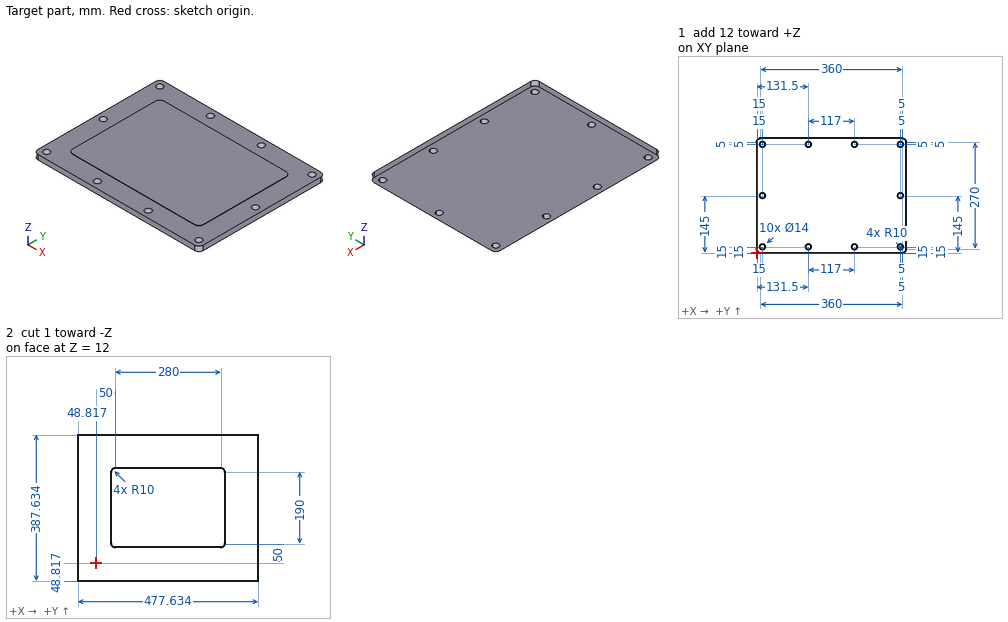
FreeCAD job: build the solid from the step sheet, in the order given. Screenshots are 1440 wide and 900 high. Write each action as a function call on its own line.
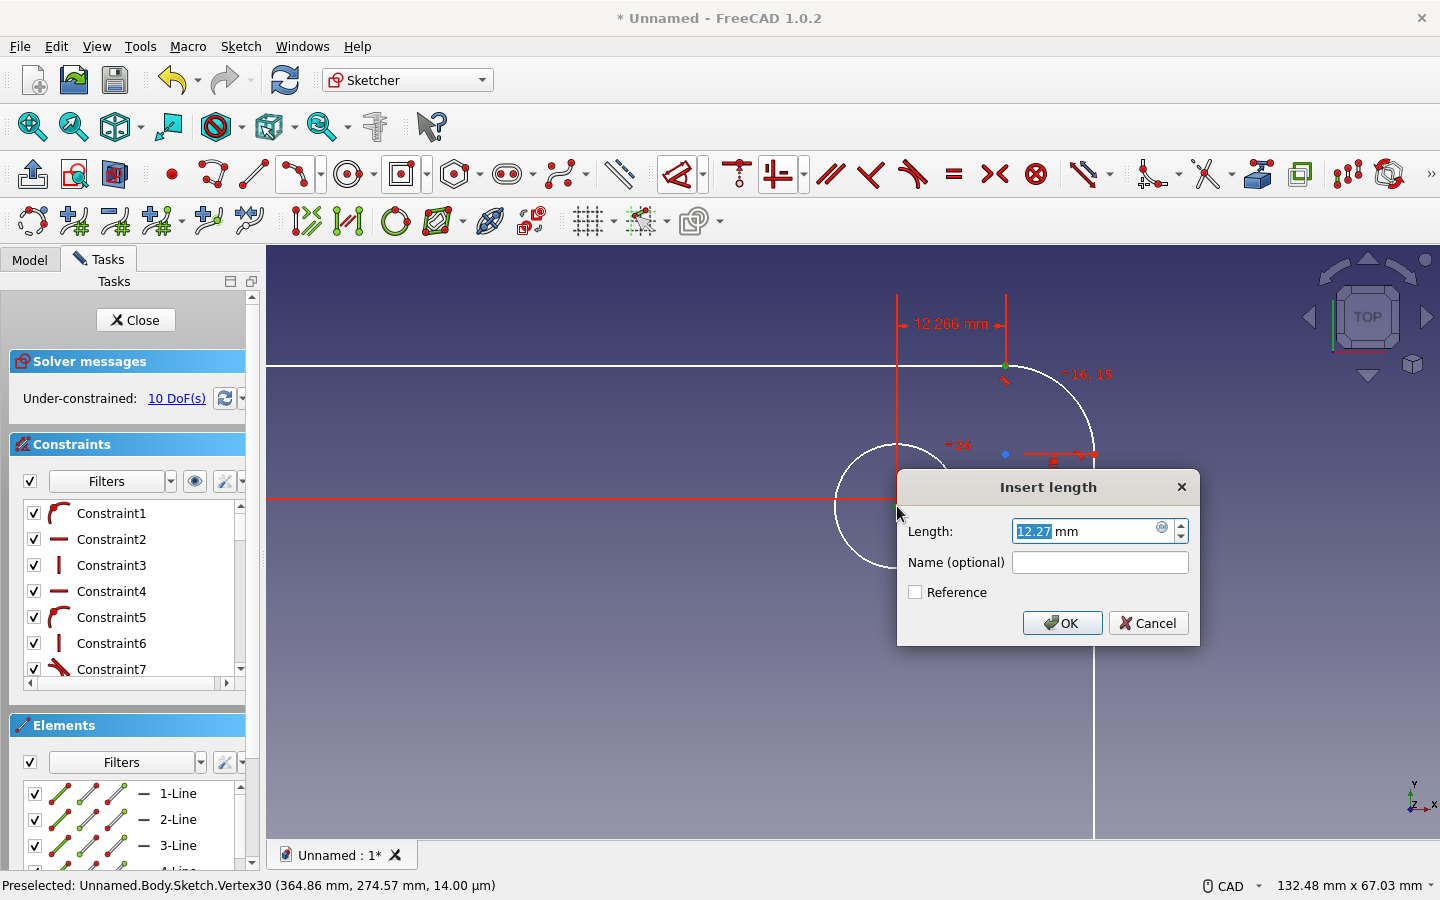
text(5)
key(Return)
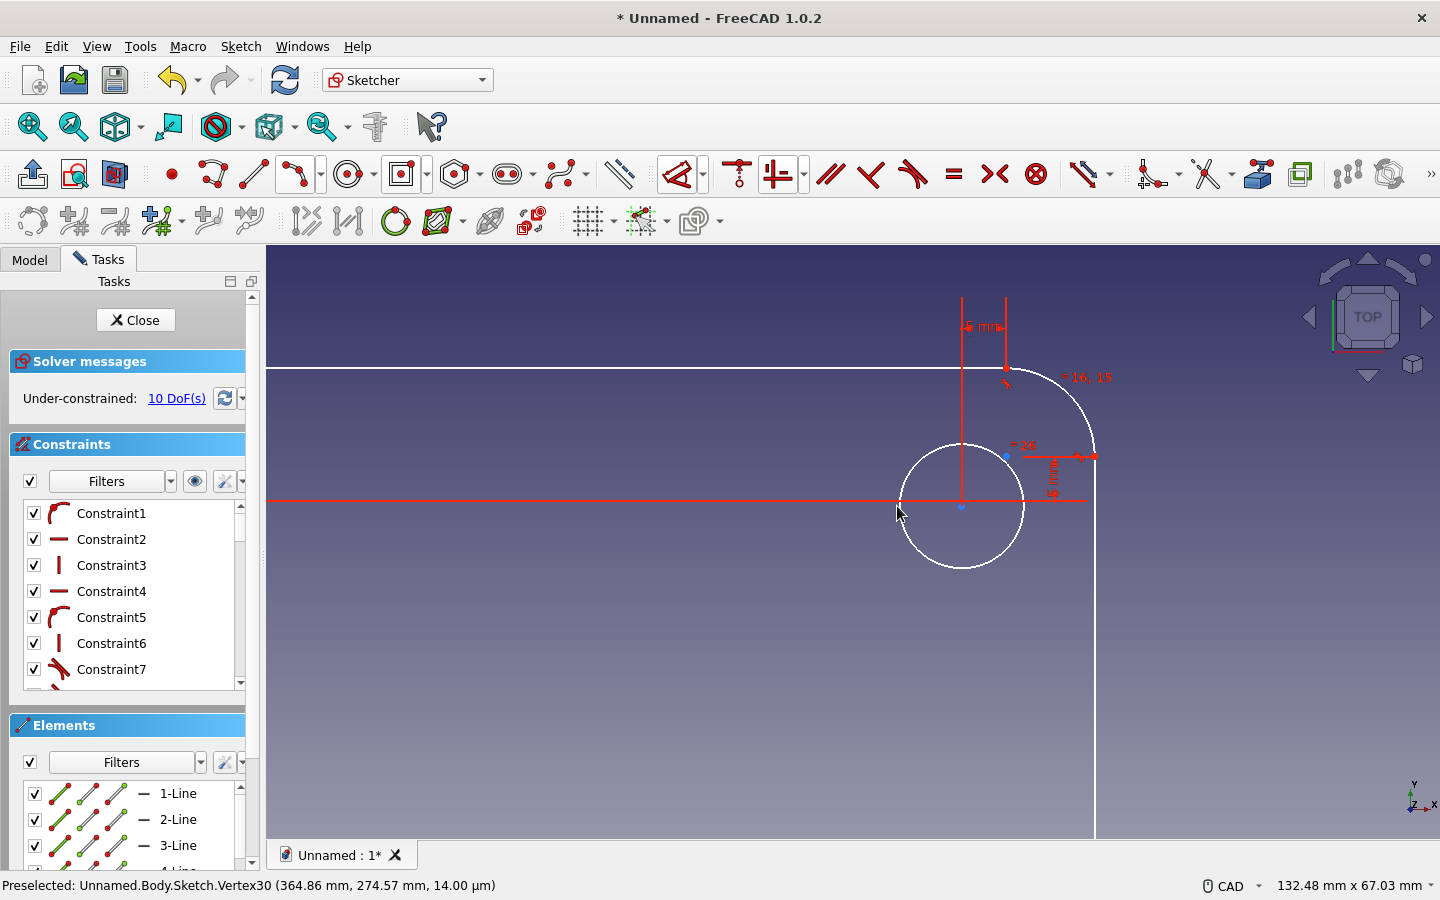
click(1095, 457)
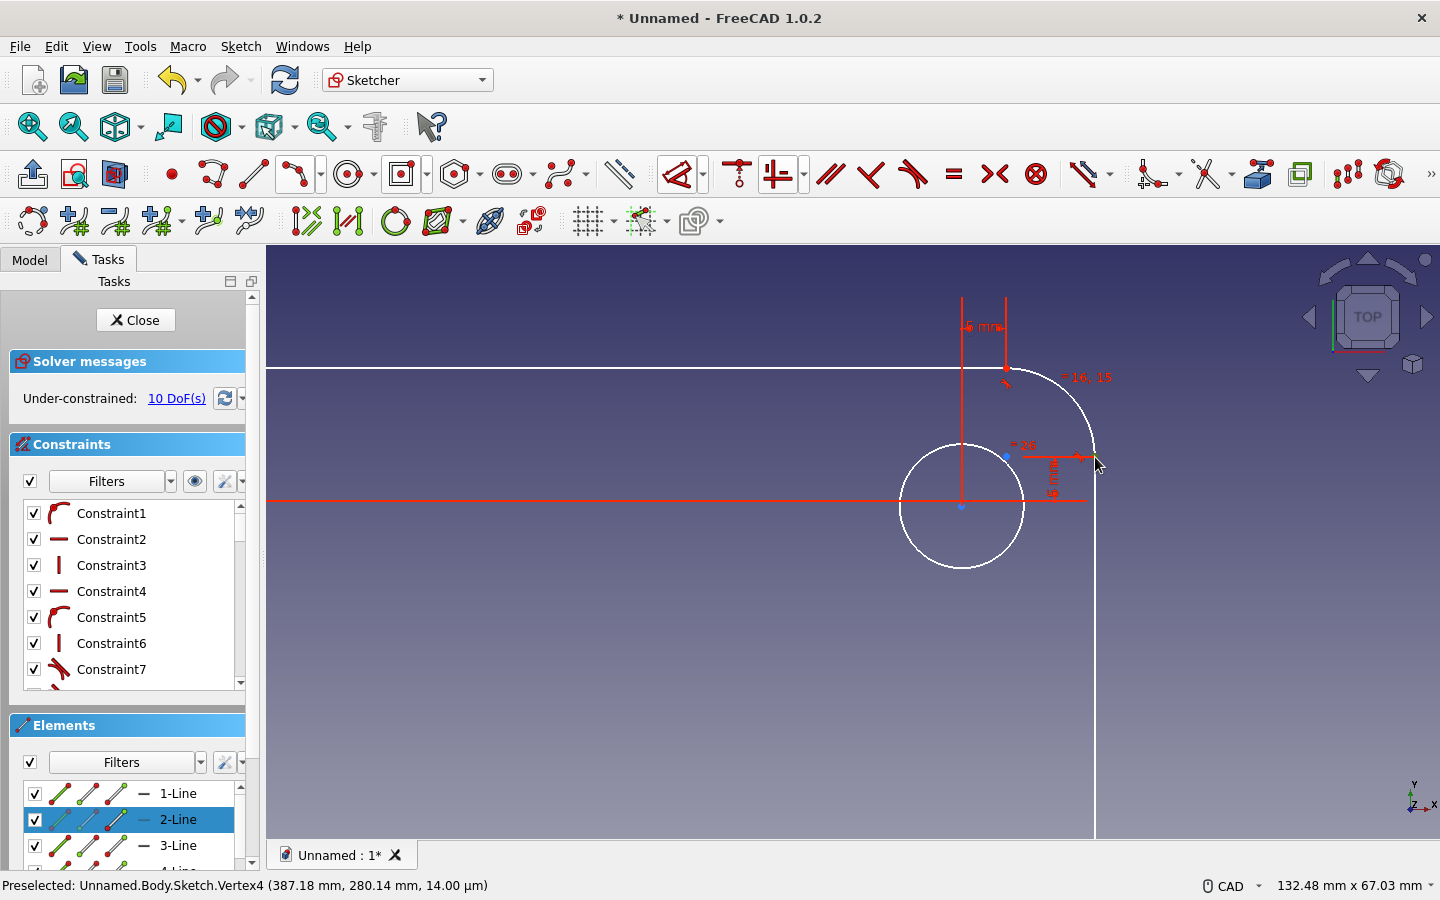
click(962, 506)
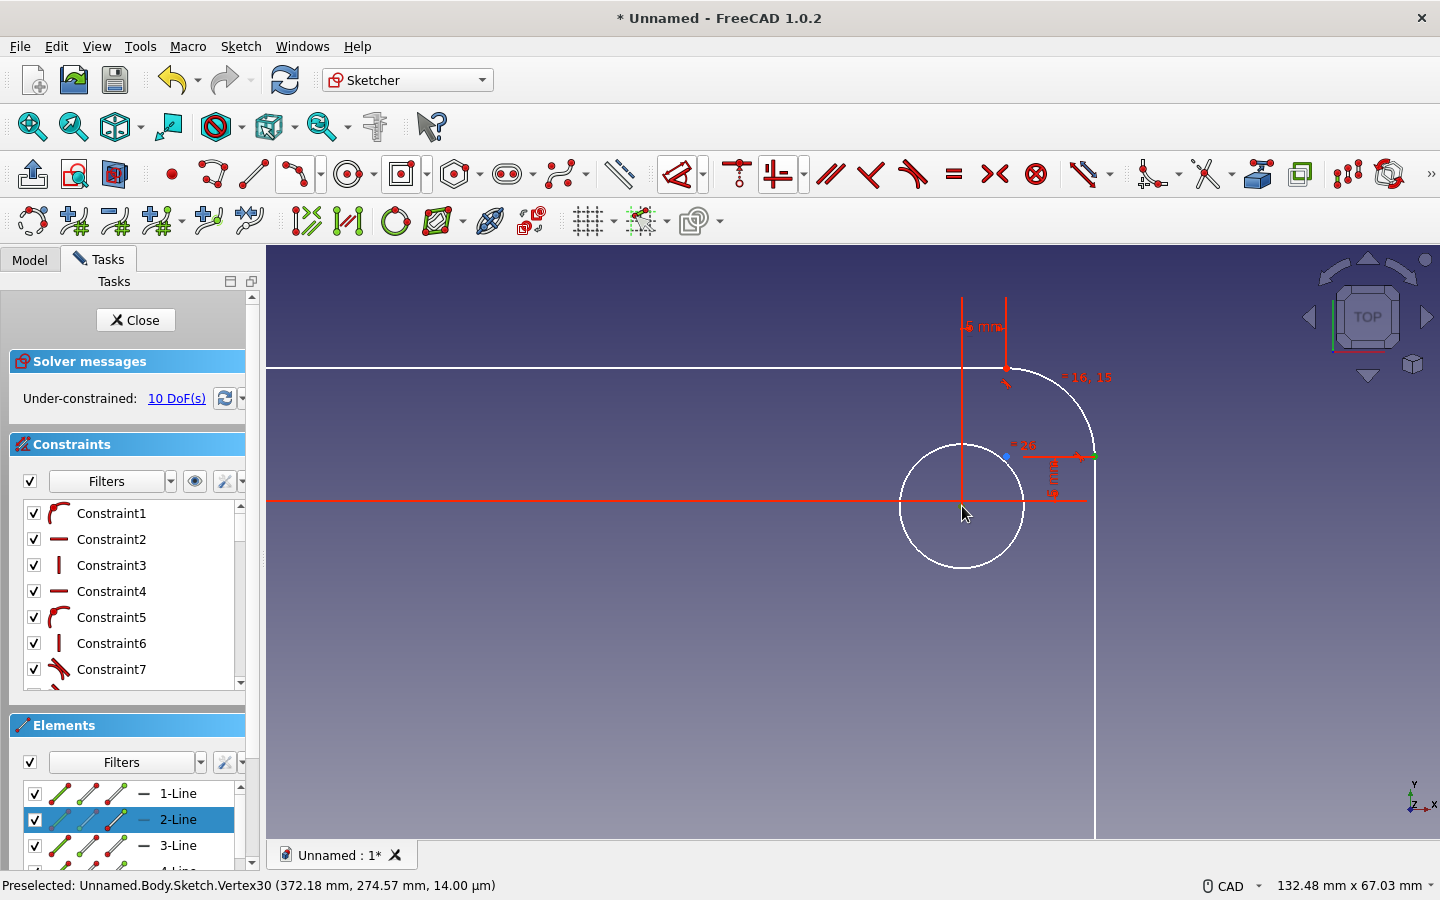
click(702, 174)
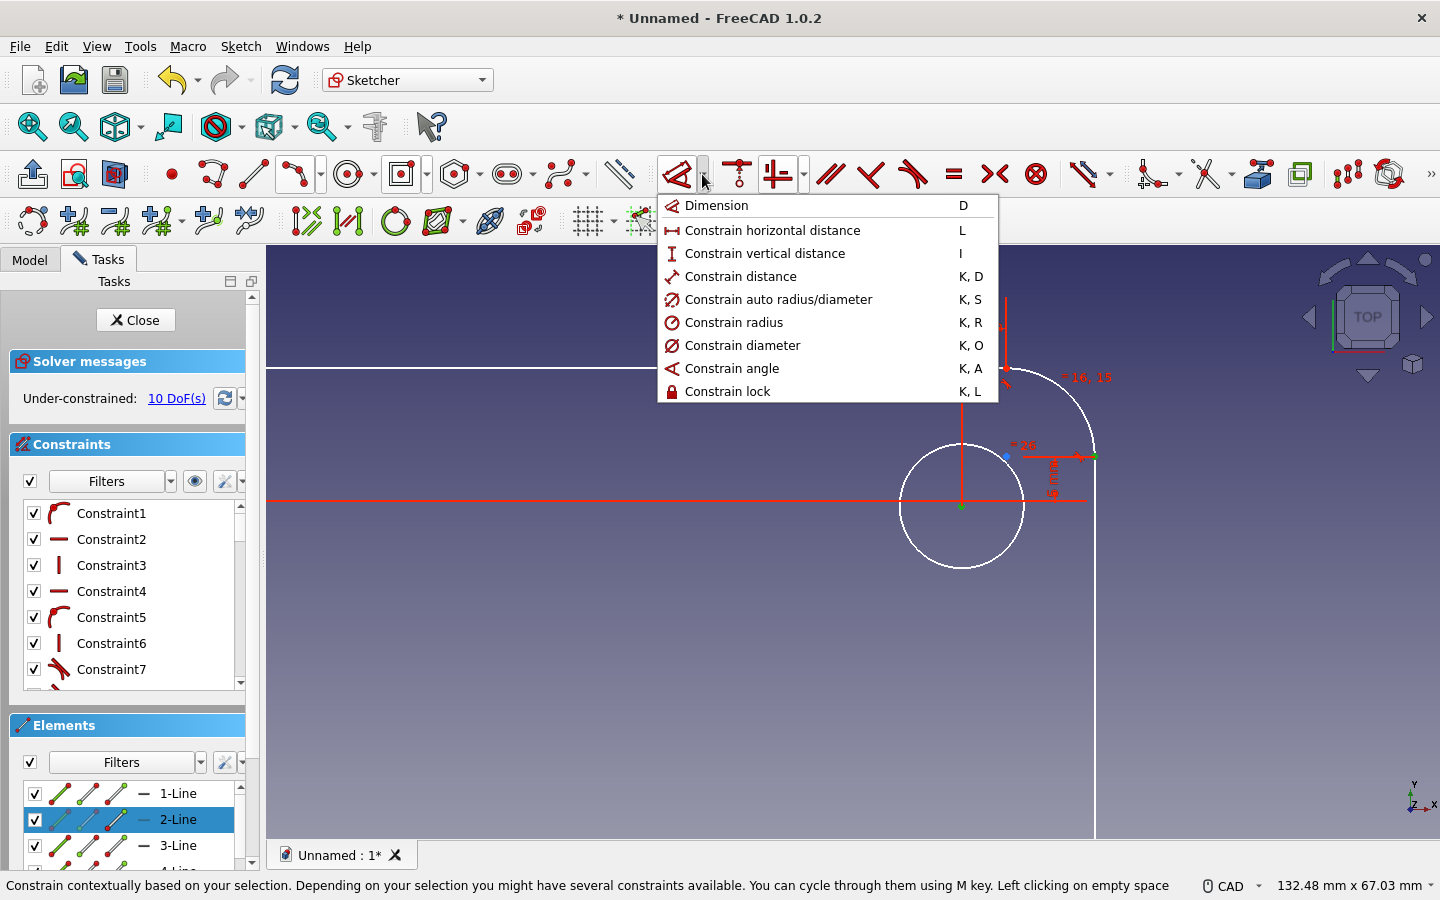
click(828, 254)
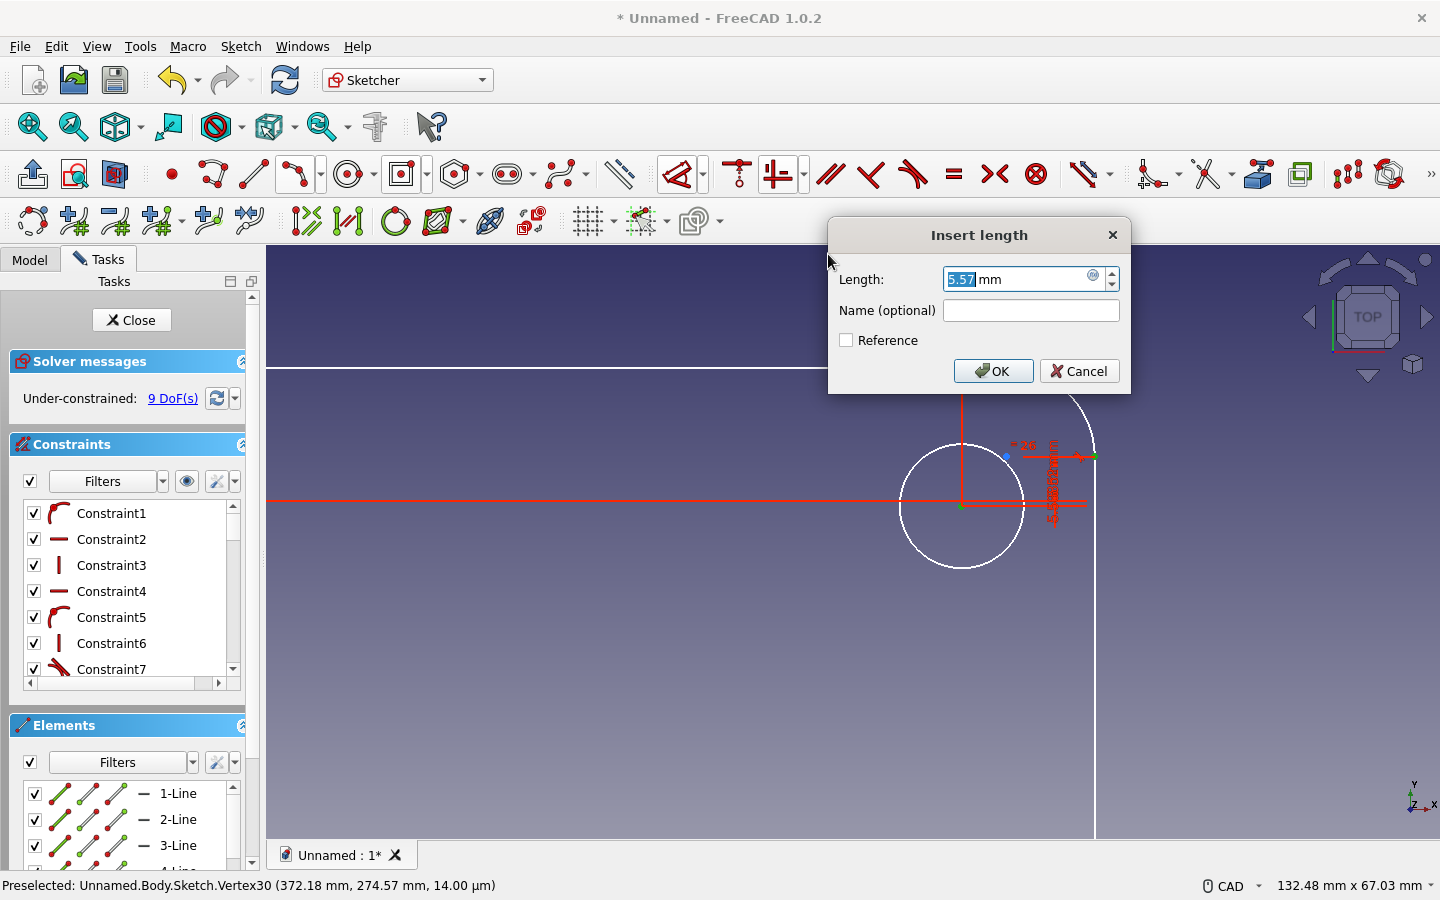
text(5)
key(Return)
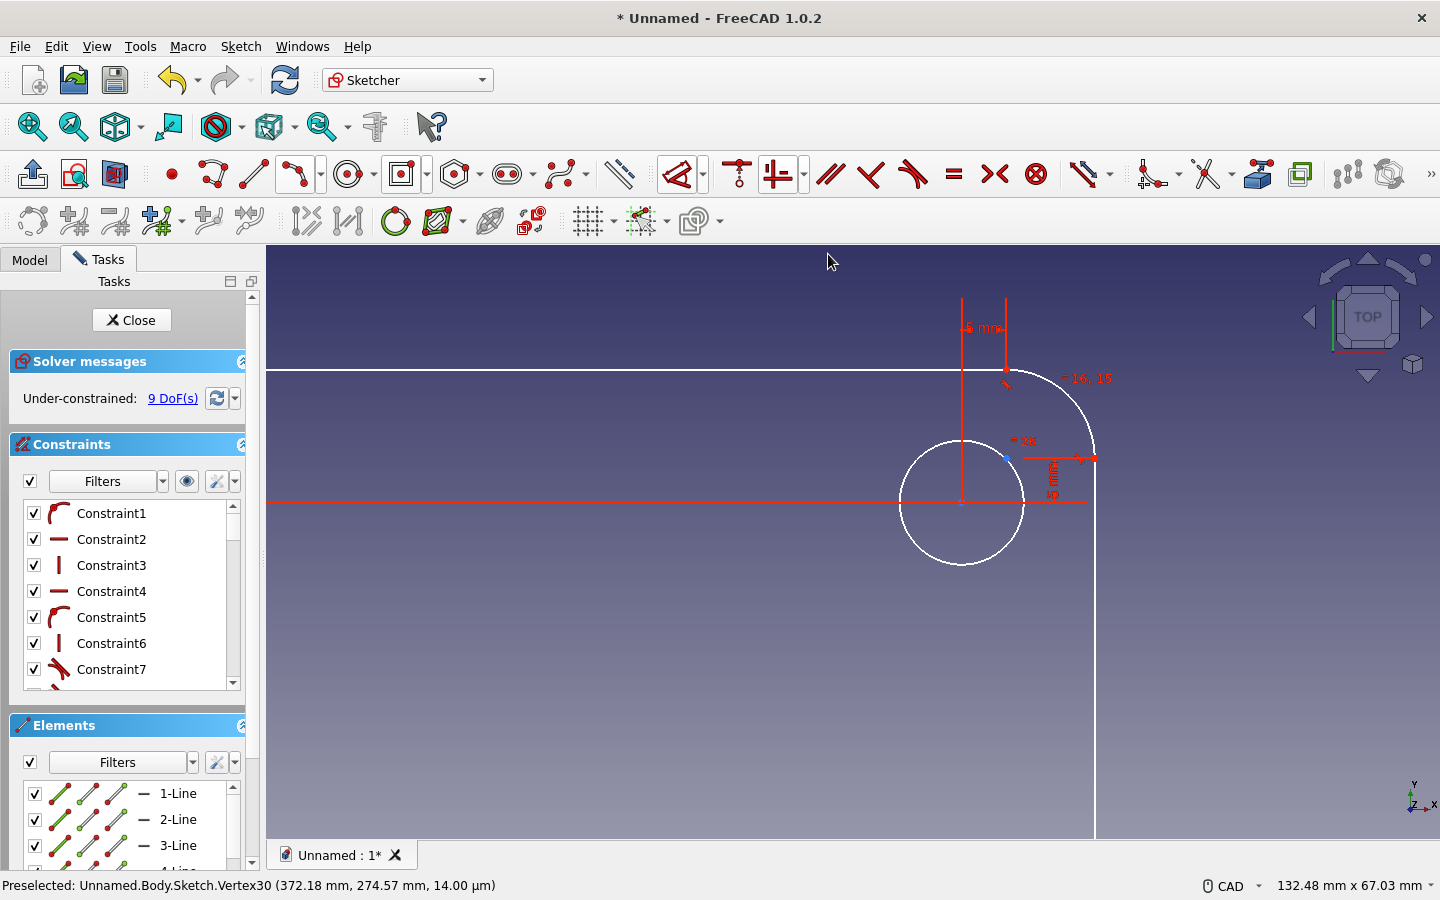
scroll(1009, 368, down, 10)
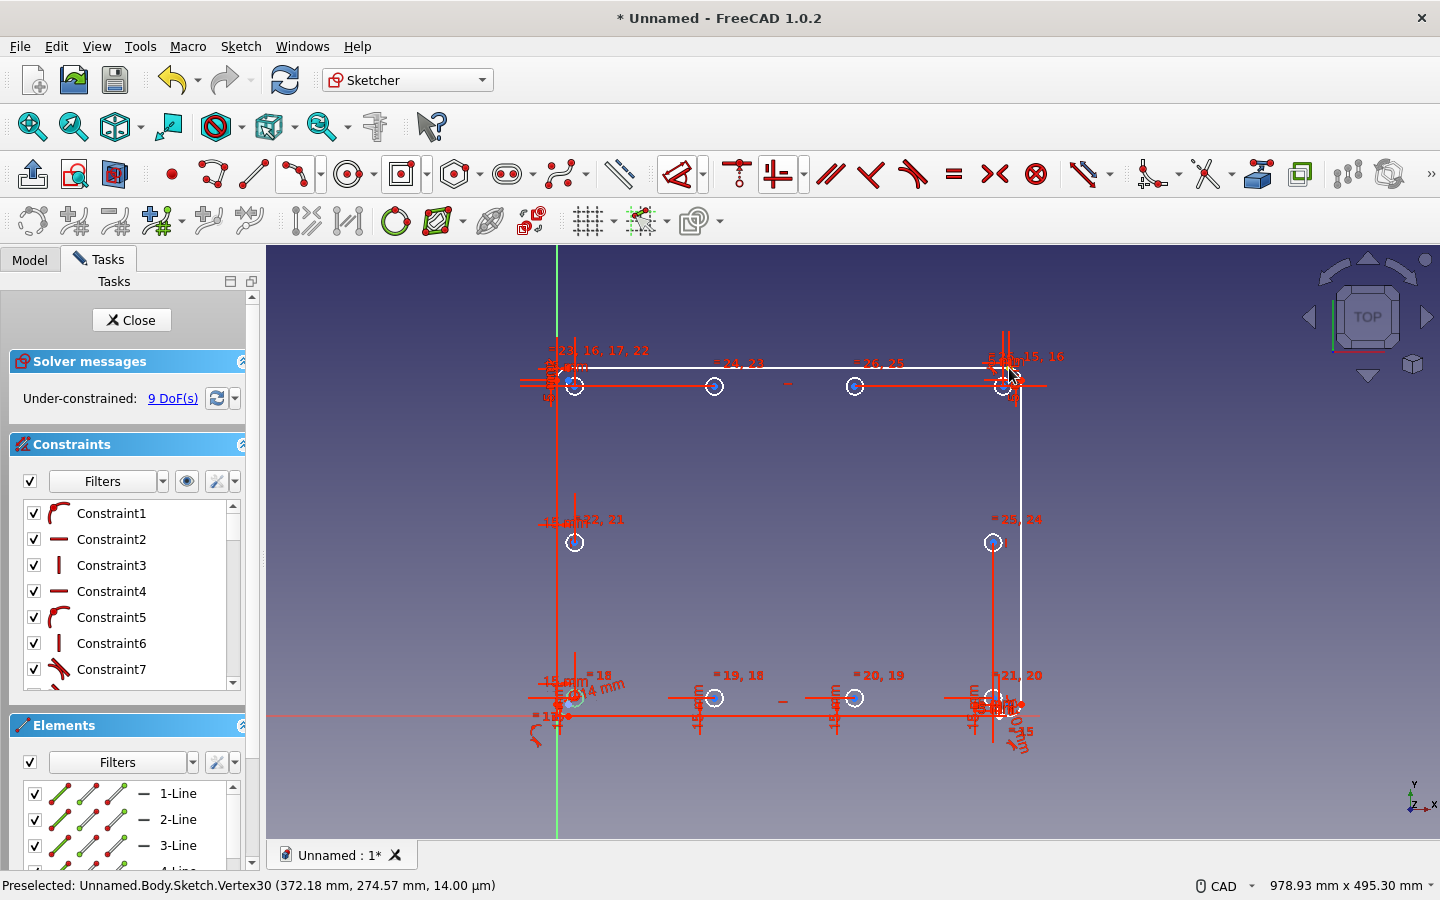
click(870, 716)